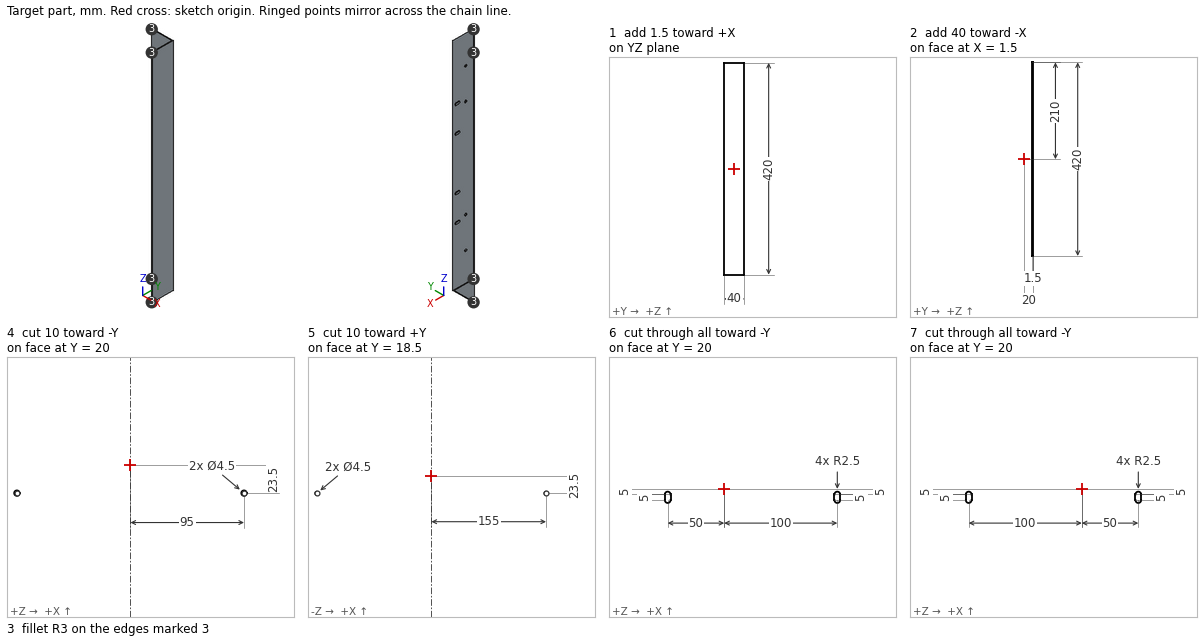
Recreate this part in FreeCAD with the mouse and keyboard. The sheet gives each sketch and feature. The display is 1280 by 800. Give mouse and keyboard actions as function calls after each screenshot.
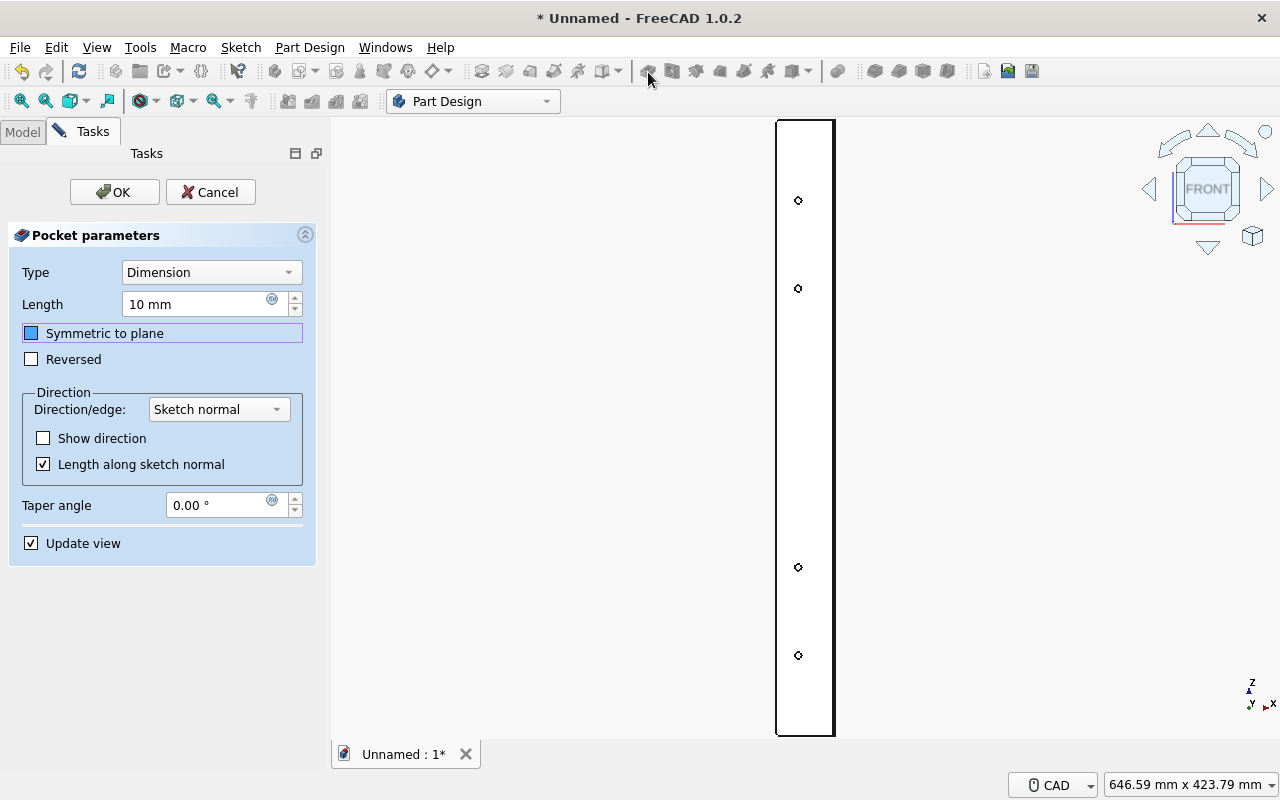
click(115, 192)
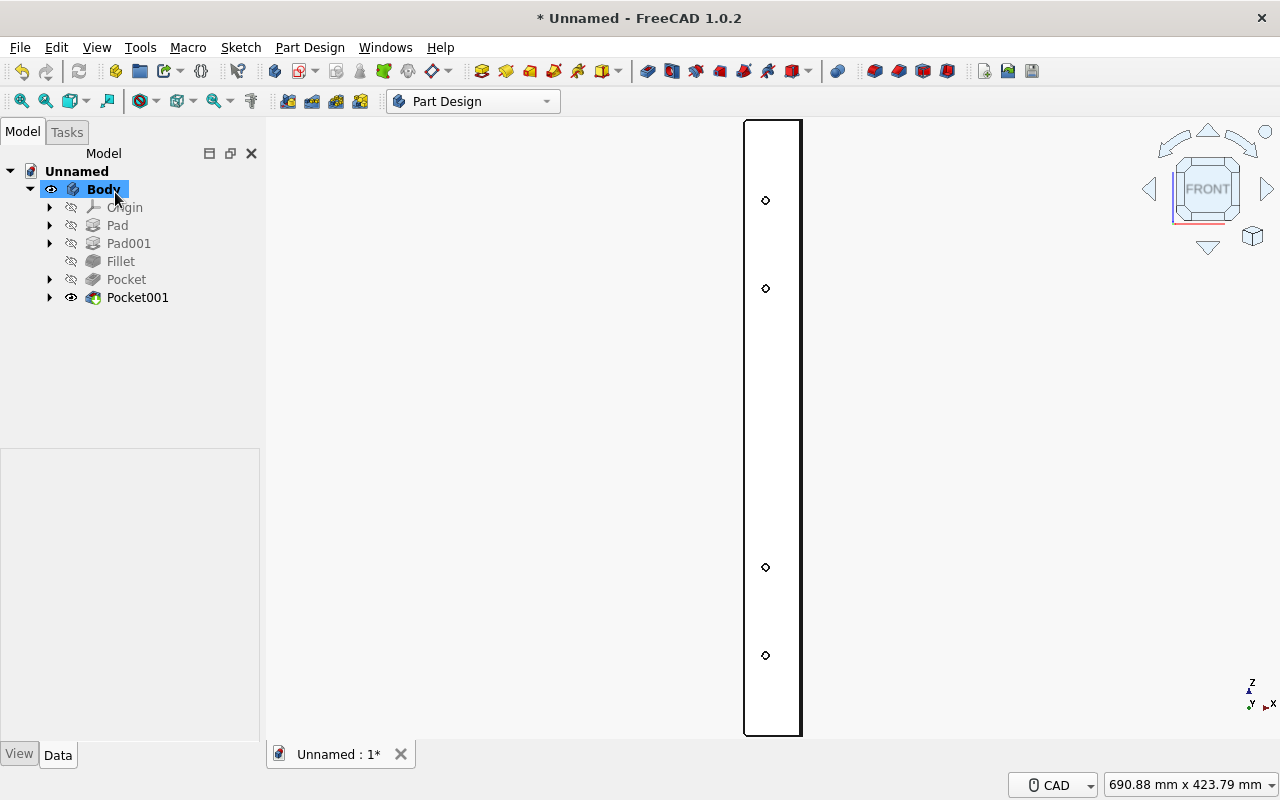
key(4)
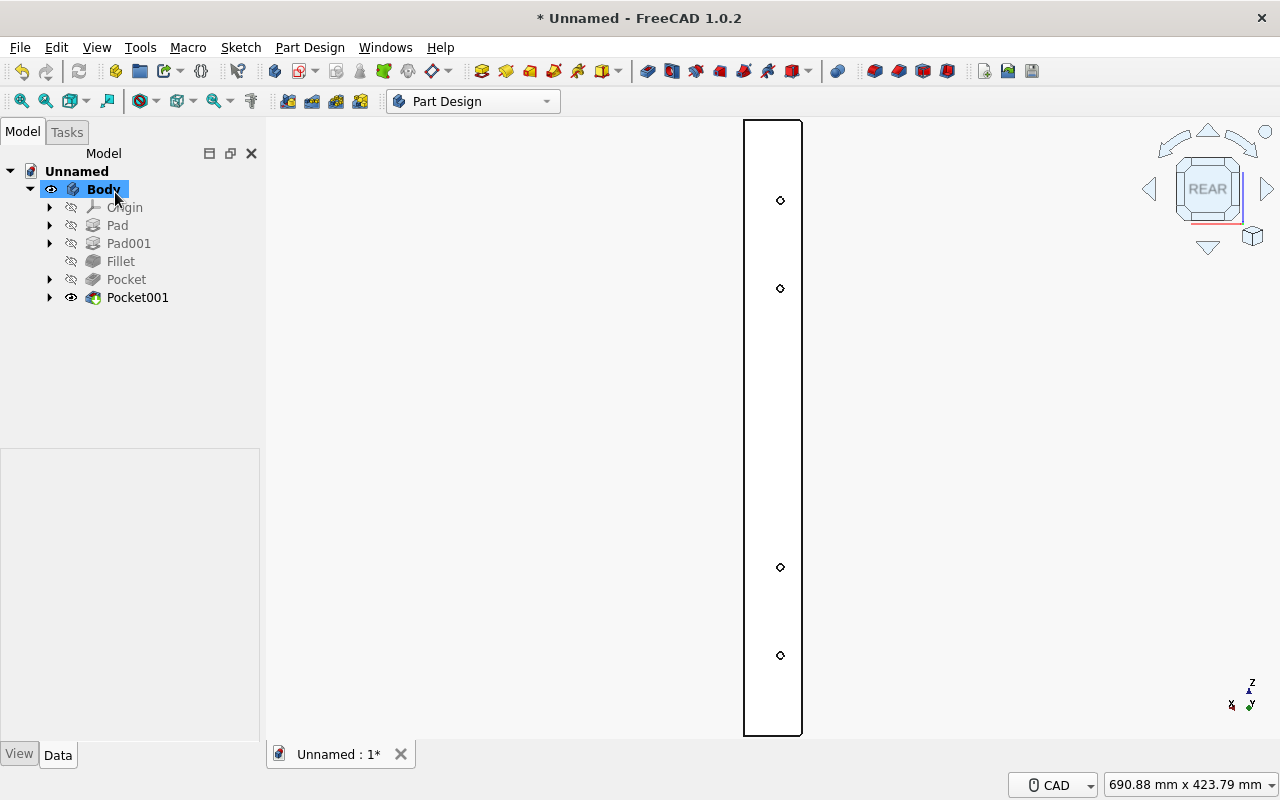
click(773, 603)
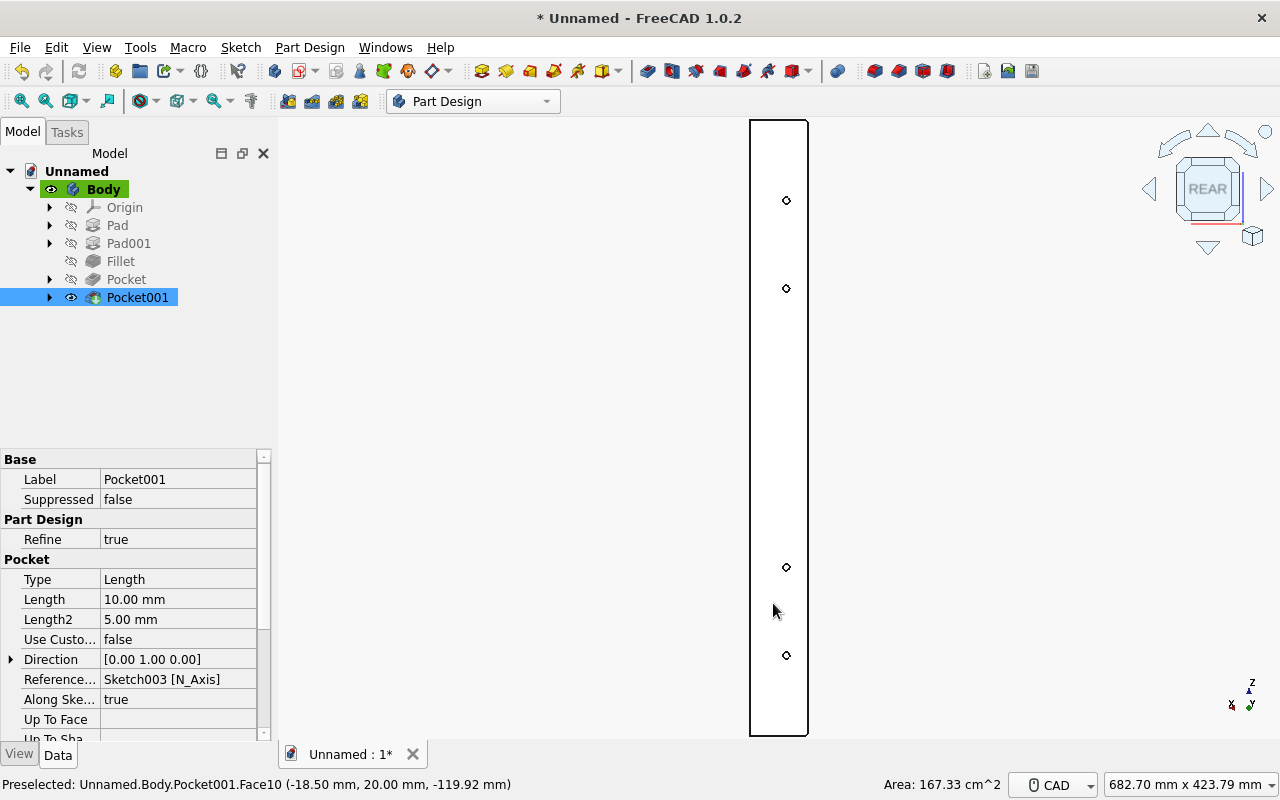
click(300, 72)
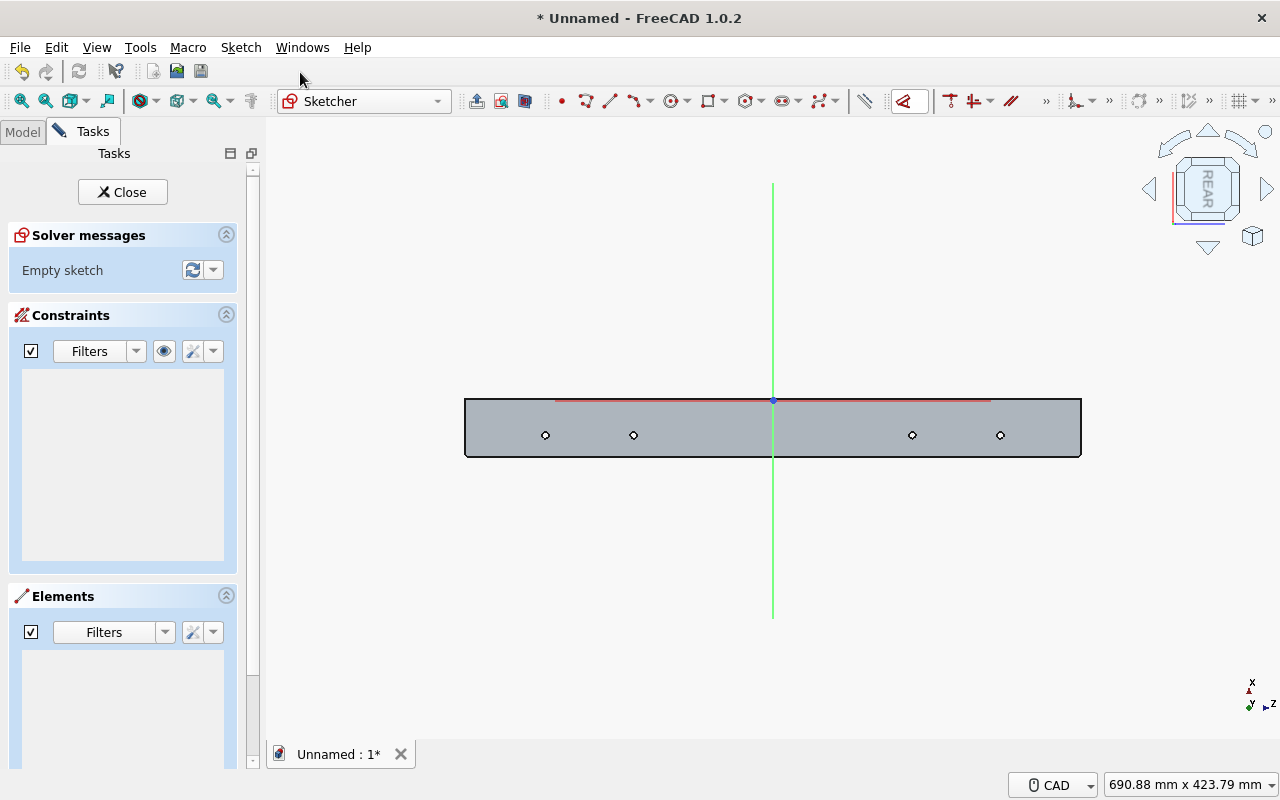
scroll(871, 400, up, 5)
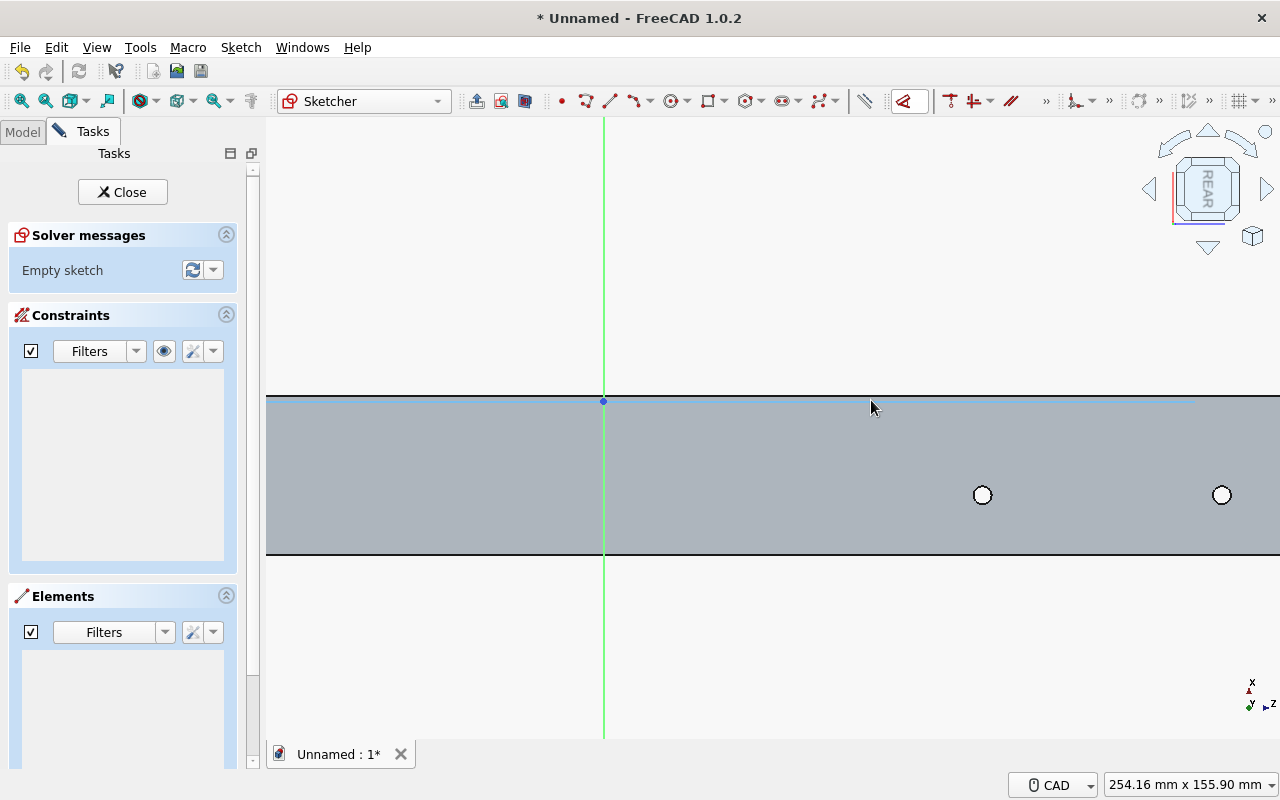
click(782, 102)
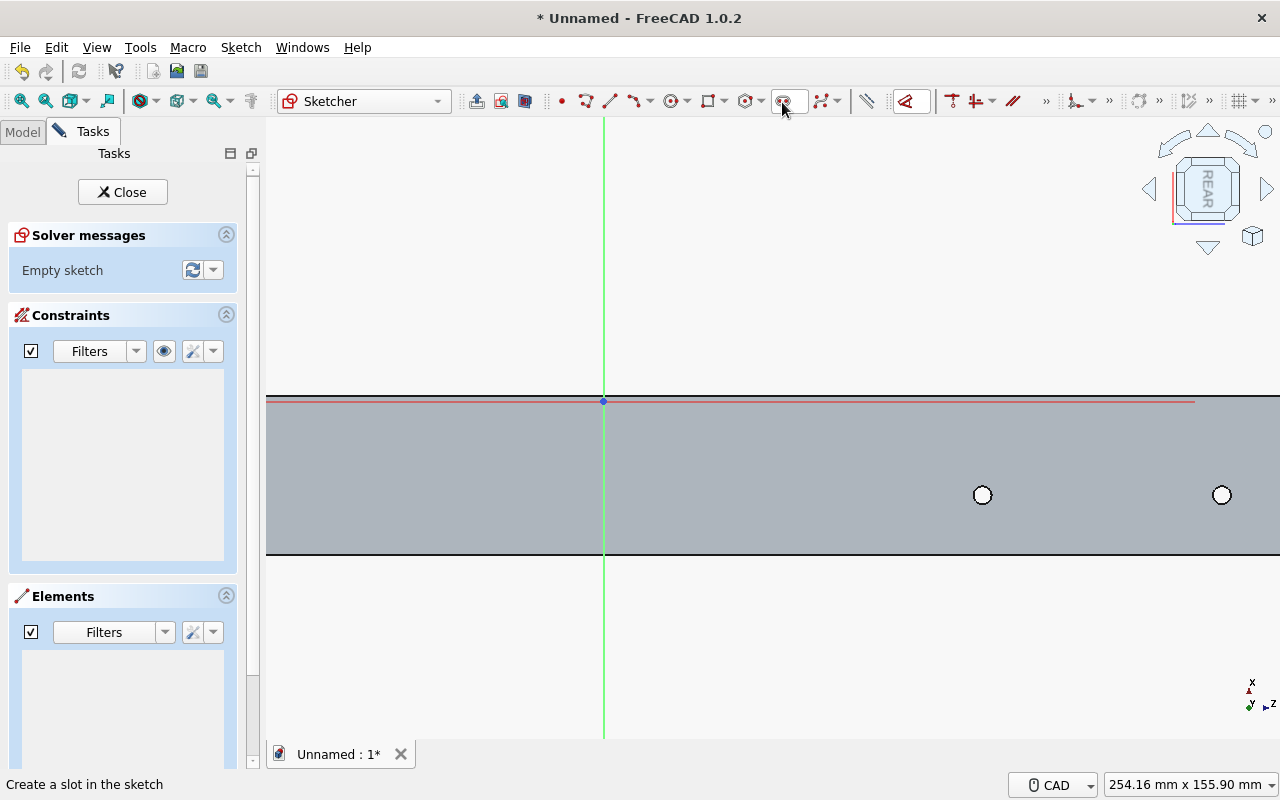
scroll(1003, 441, up, 5)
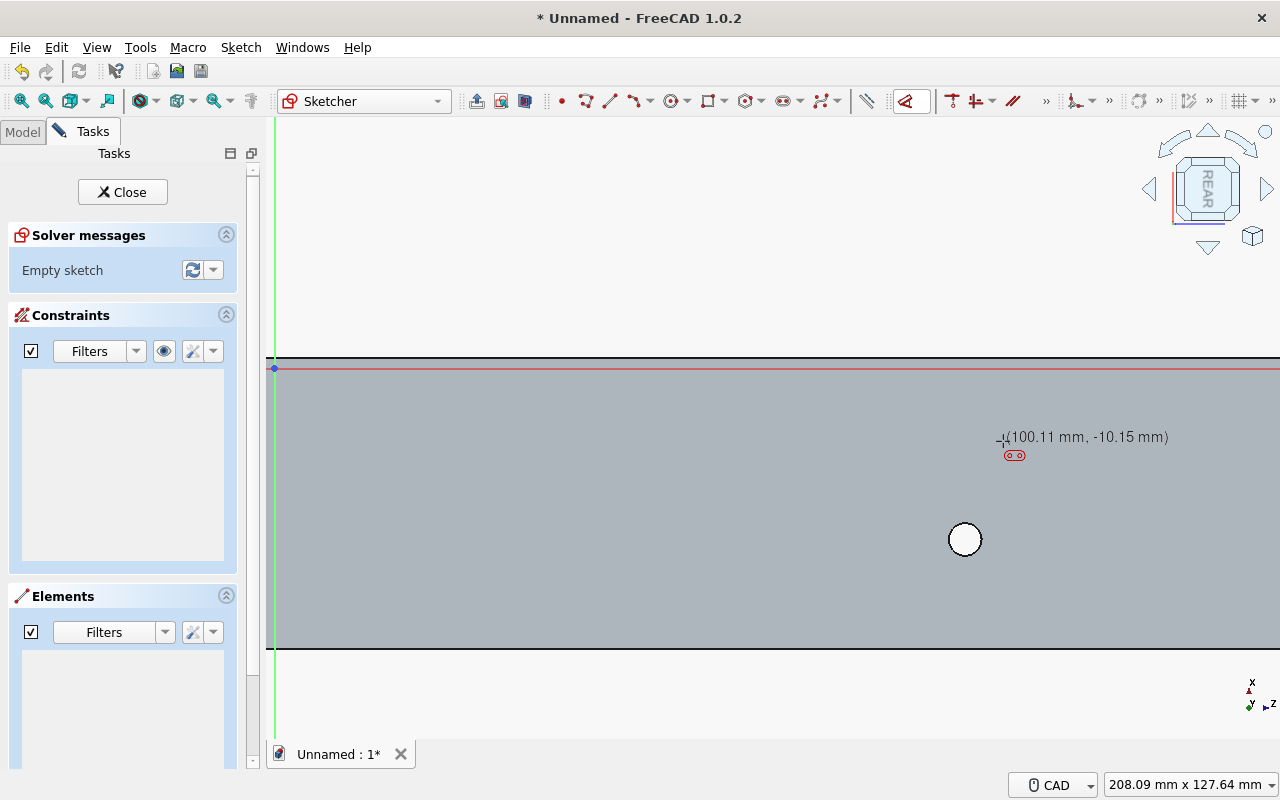
click(1001, 441)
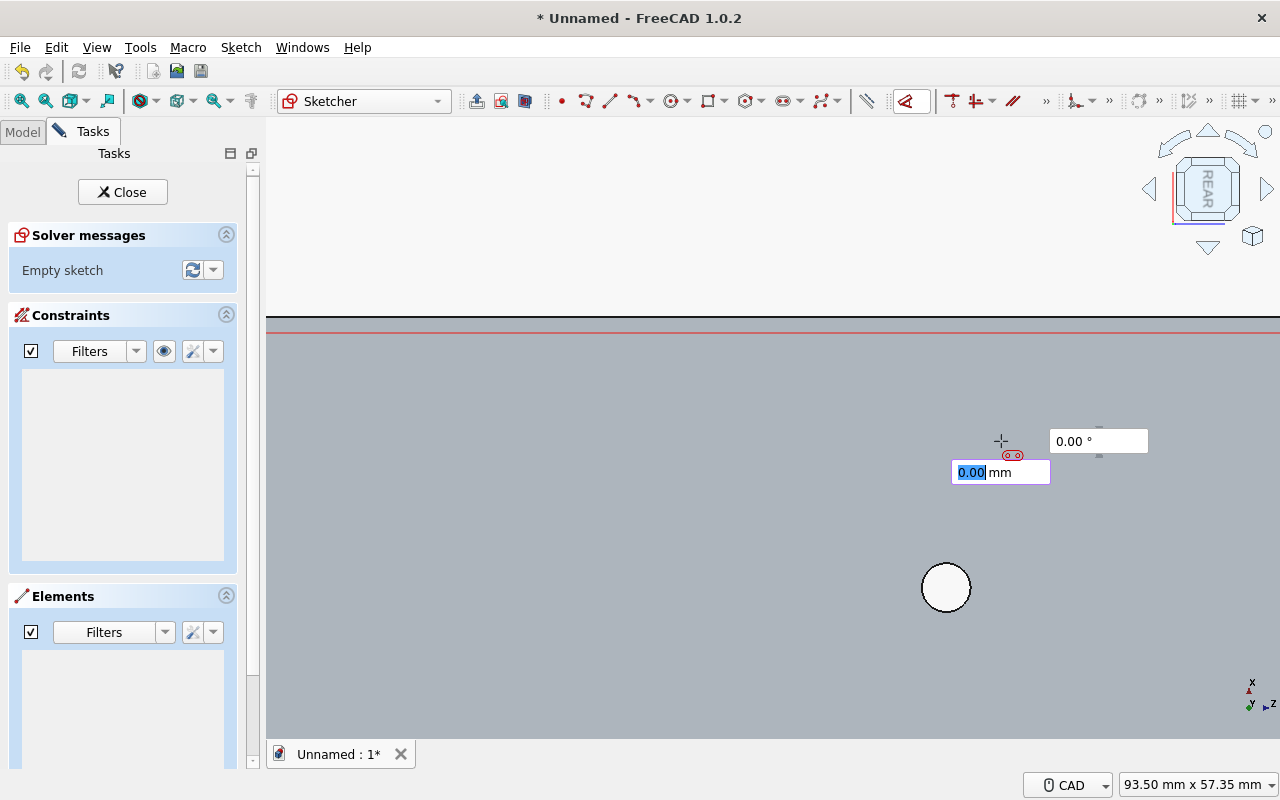
click(1001, 387)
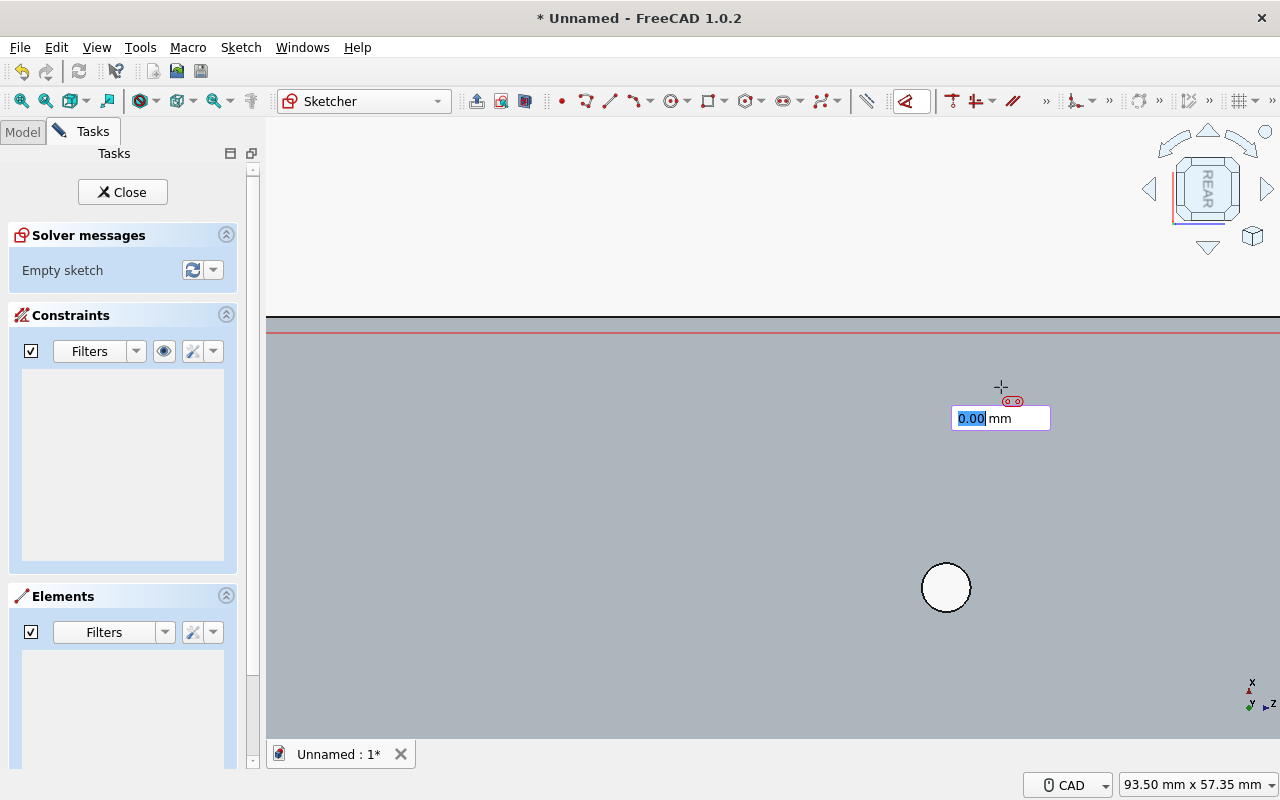
click(973, 414)